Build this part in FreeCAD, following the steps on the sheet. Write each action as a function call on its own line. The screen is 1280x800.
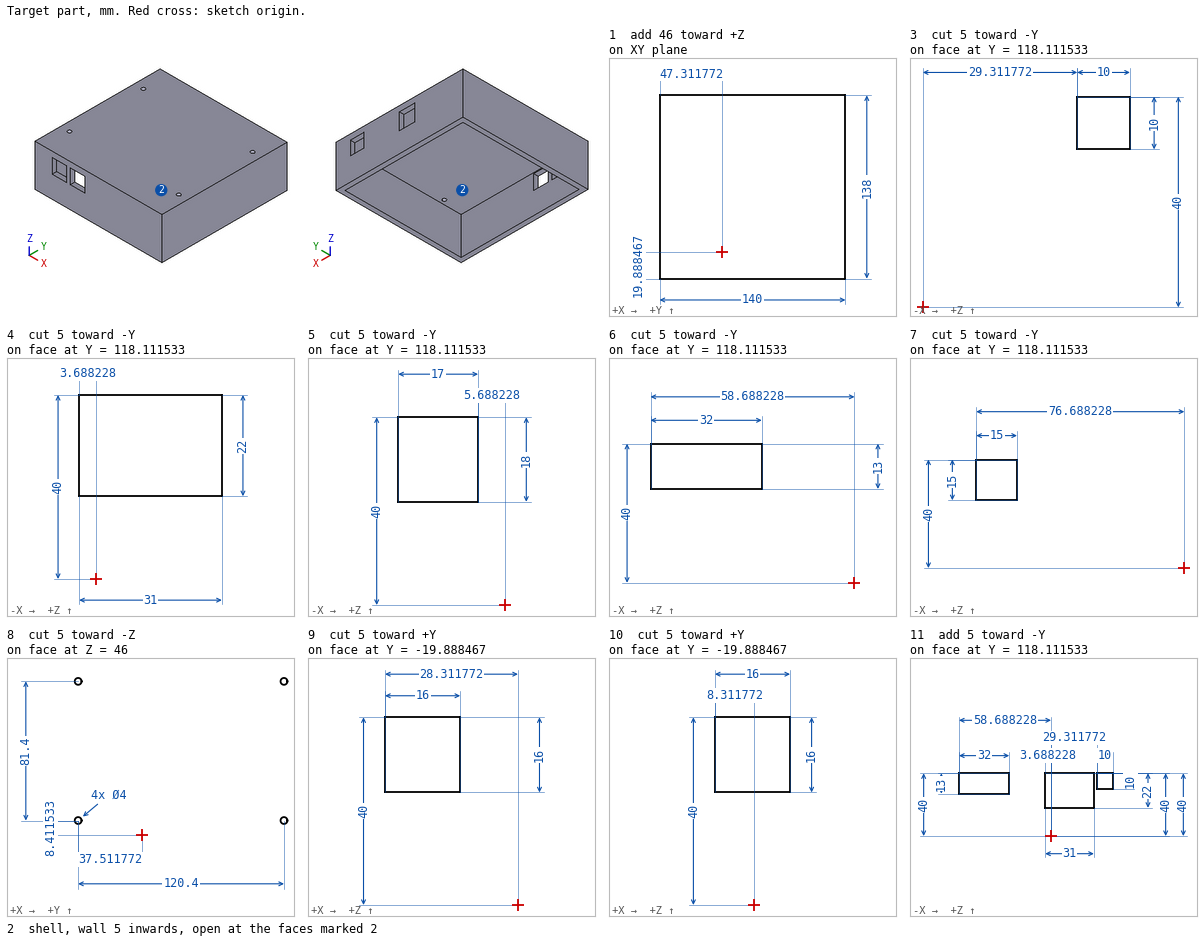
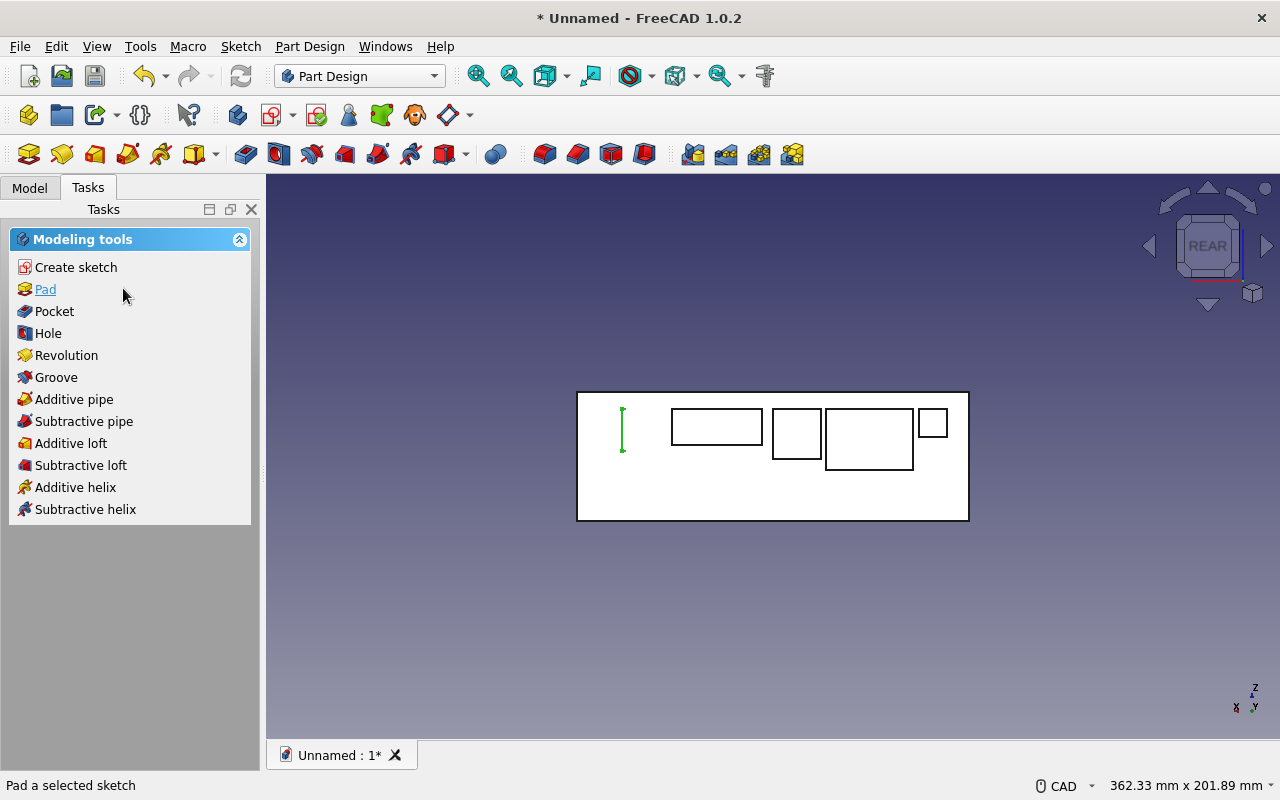
click(246, 154)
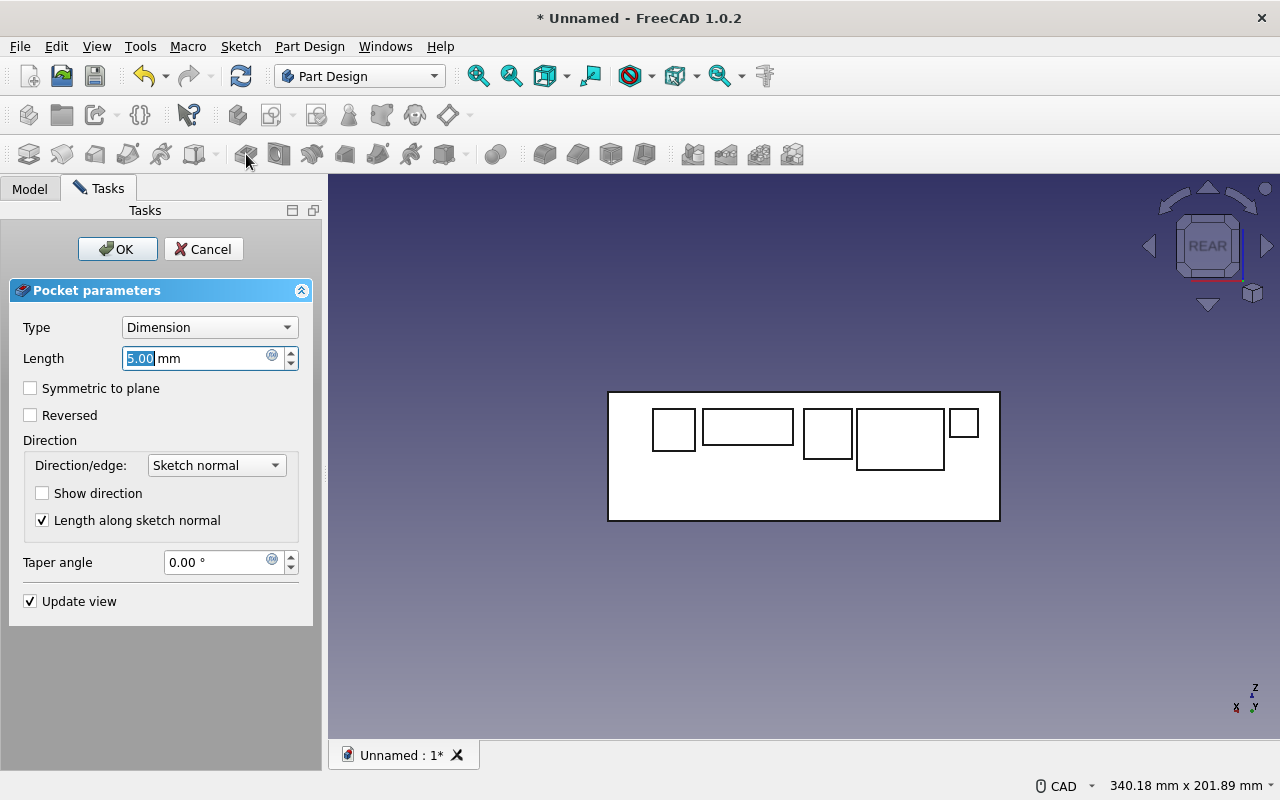
text(5)
key(Tab)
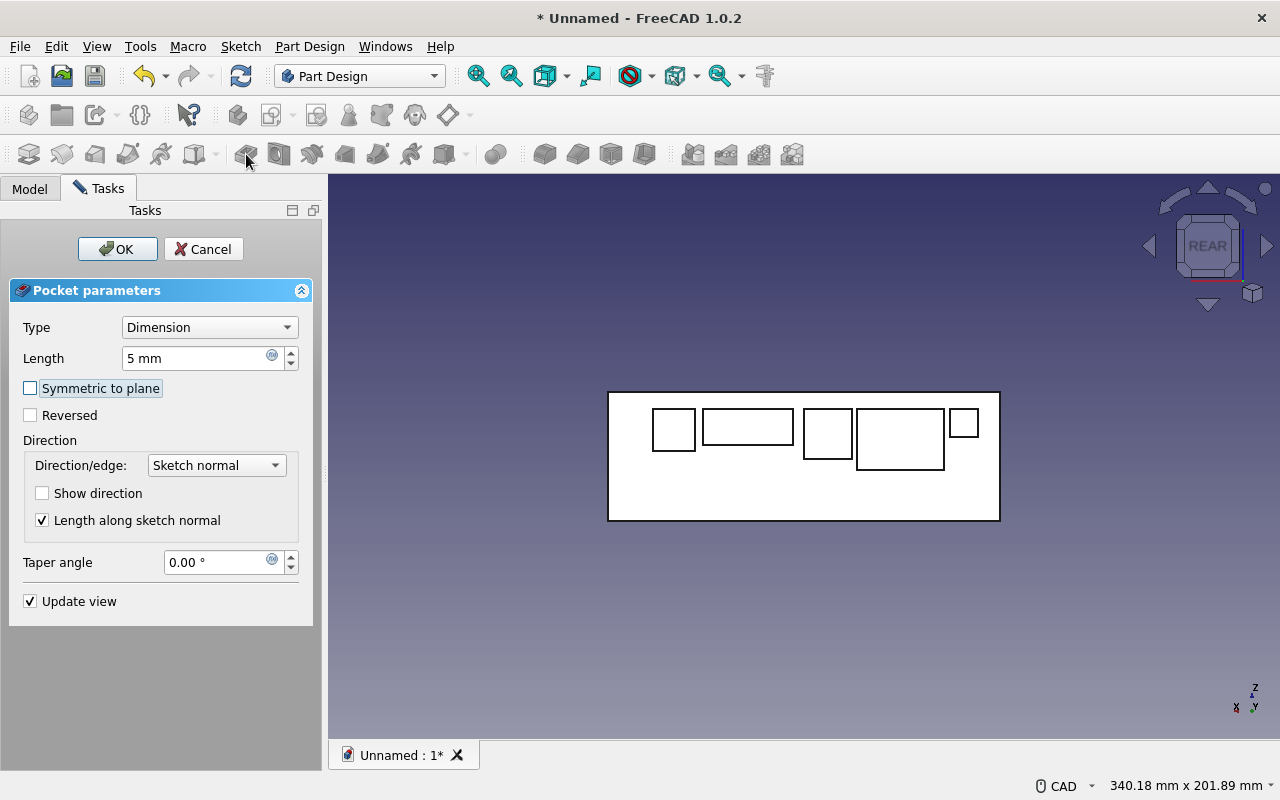
click(118, 249)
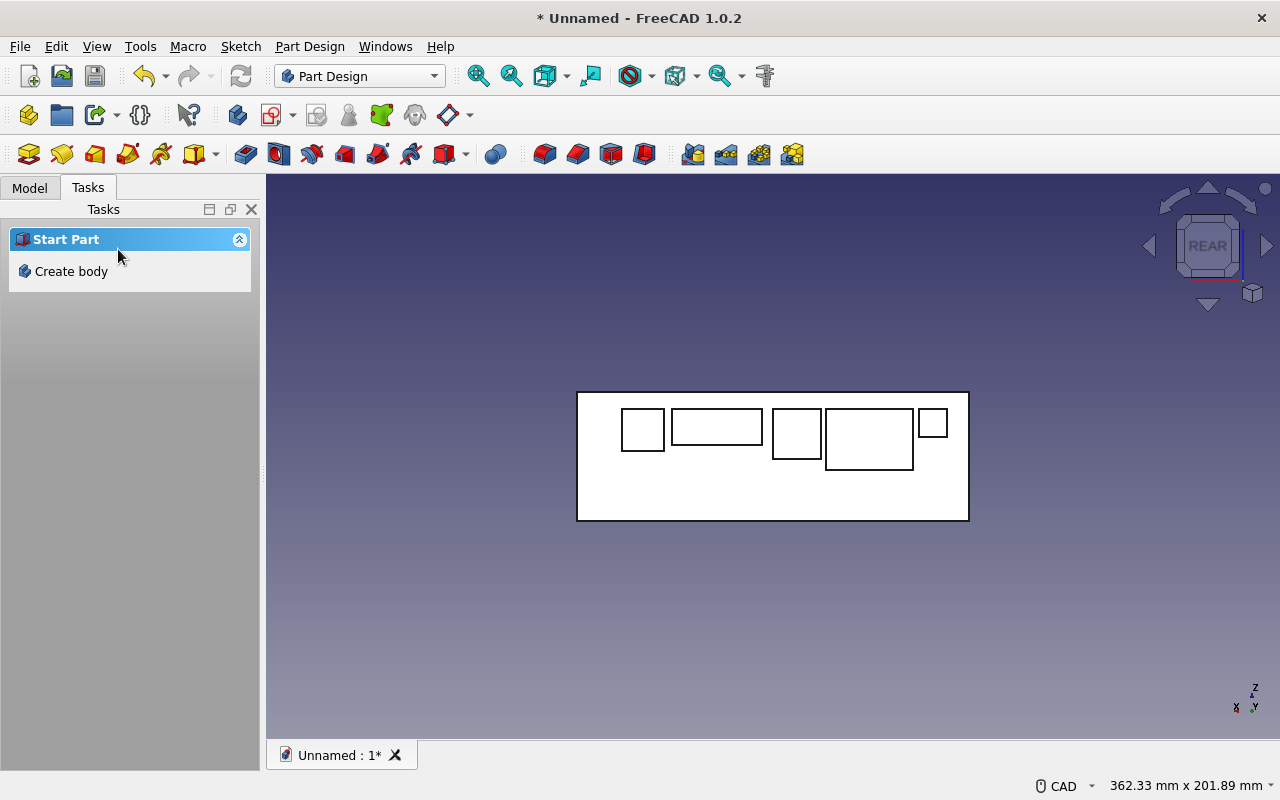
click(479, 76)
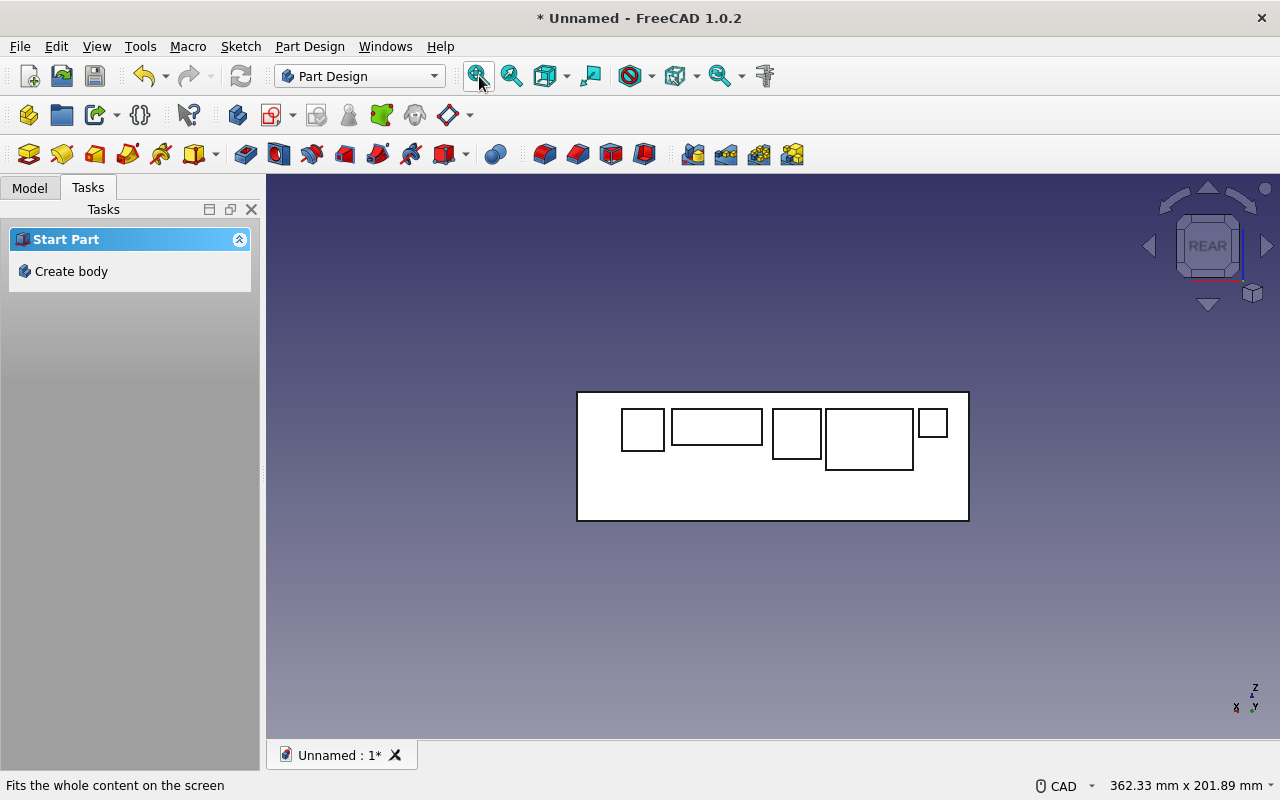
key(0)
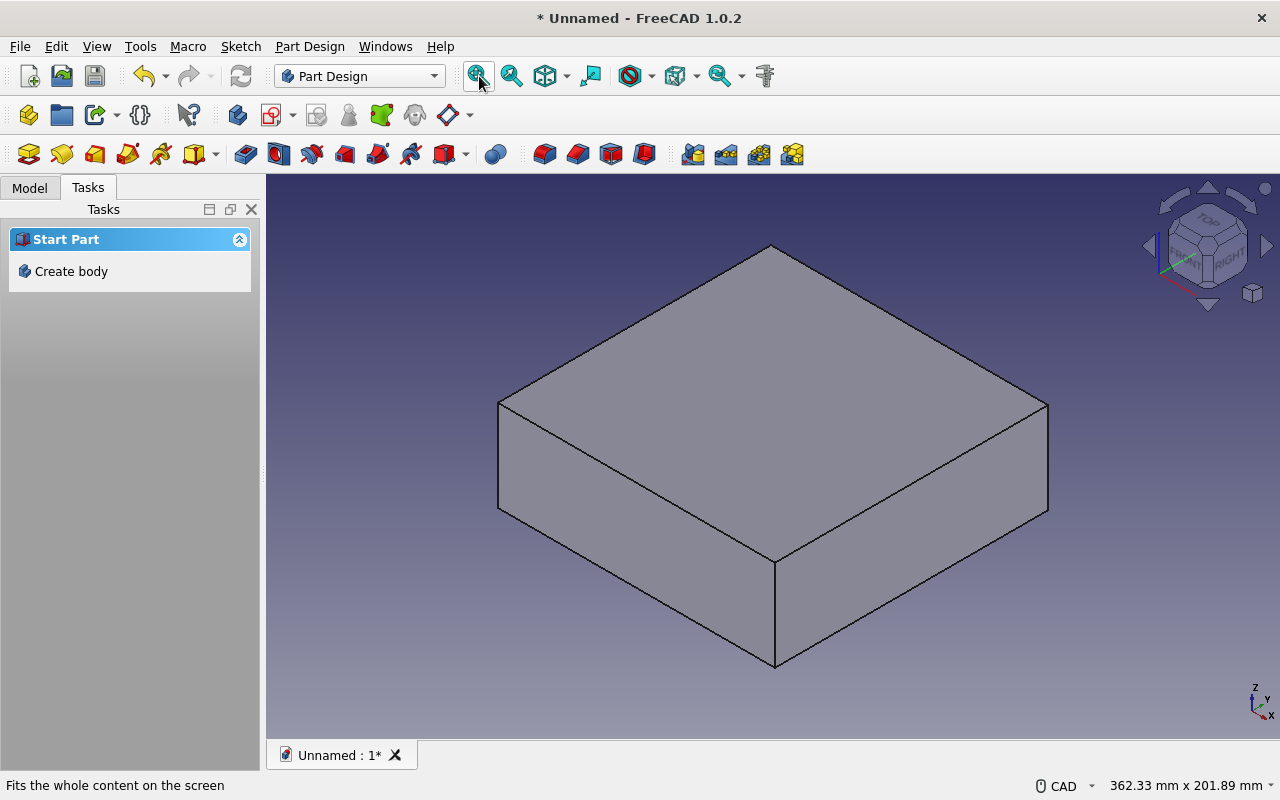
click(773, 403)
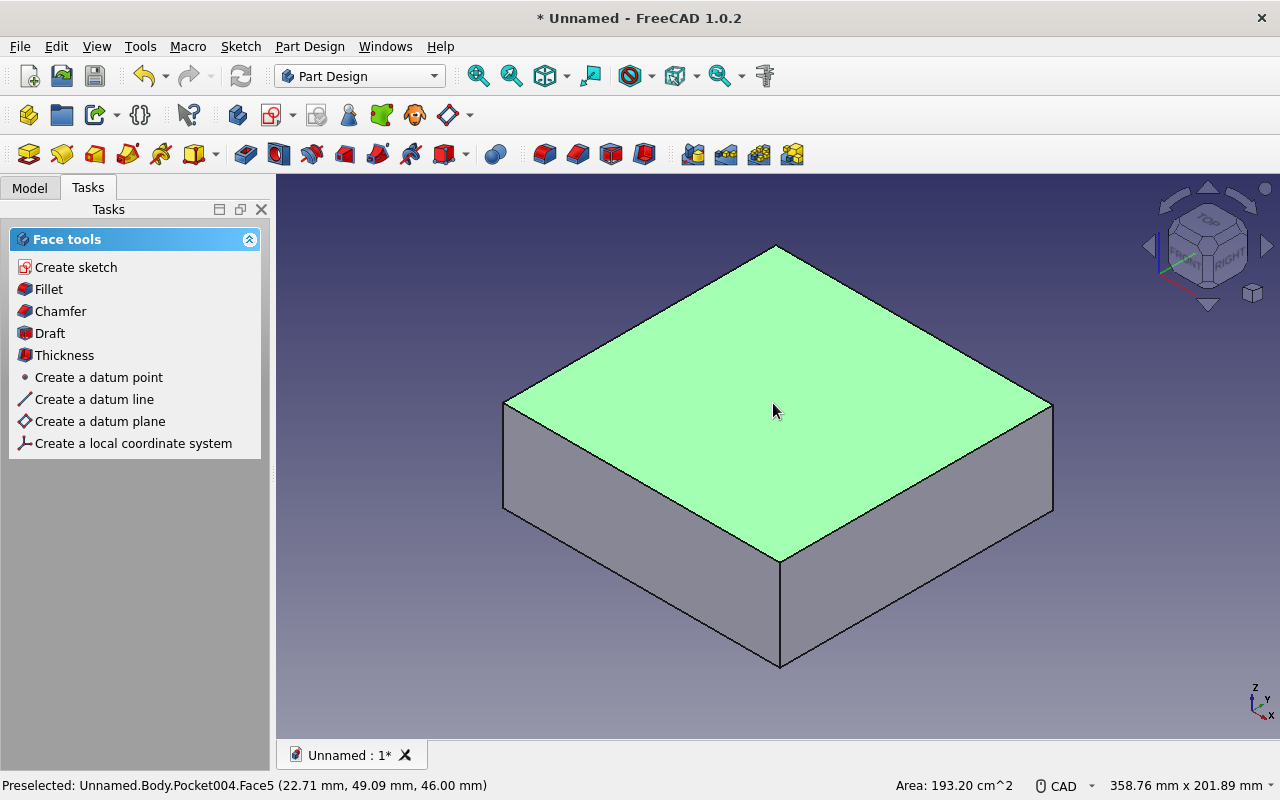
click(270, 116)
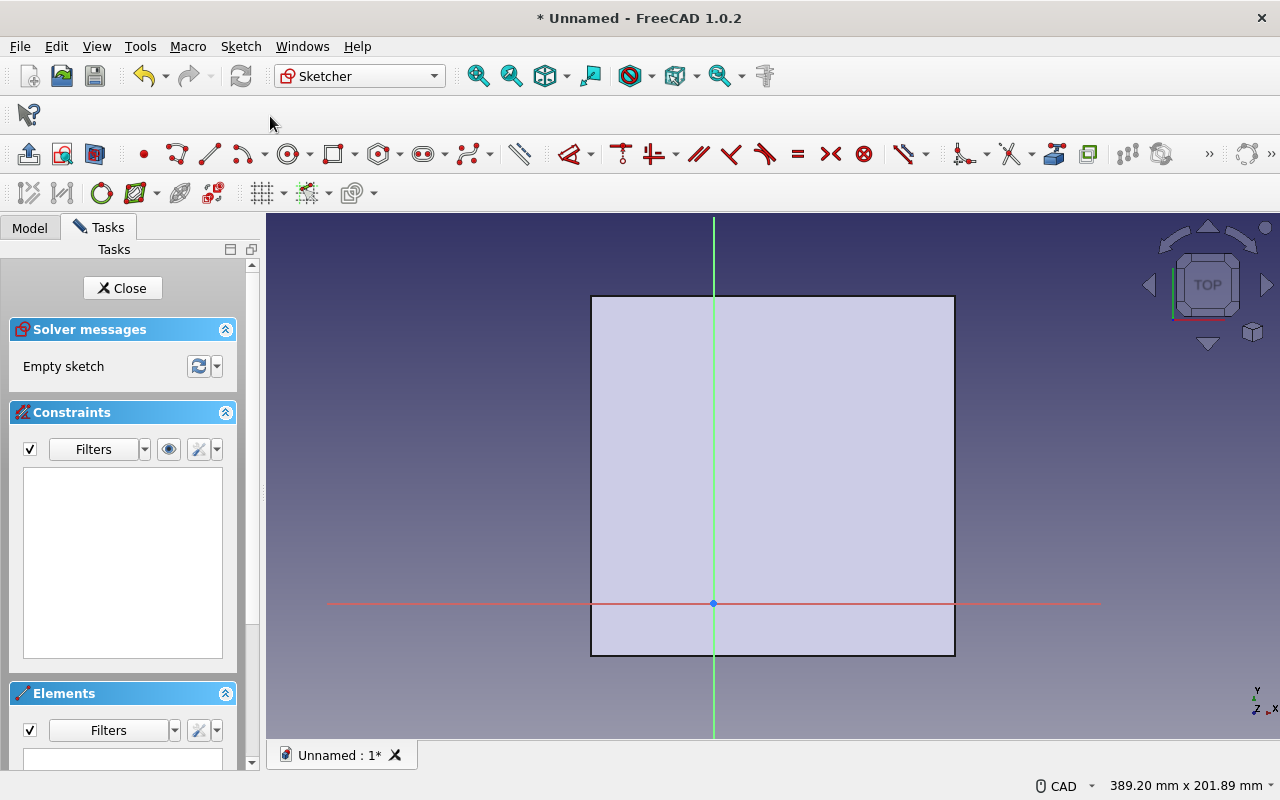
scroll(912, 501, up, 2)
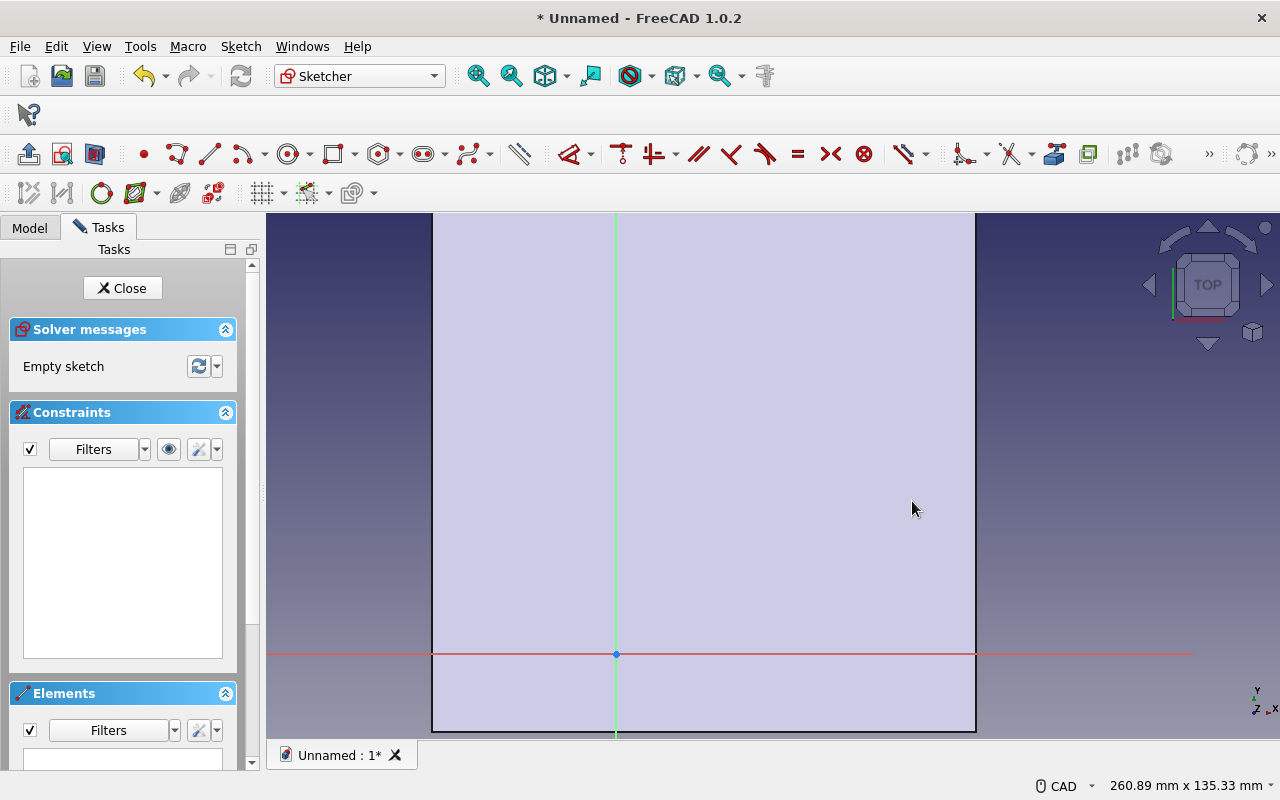
key(g)
key(c)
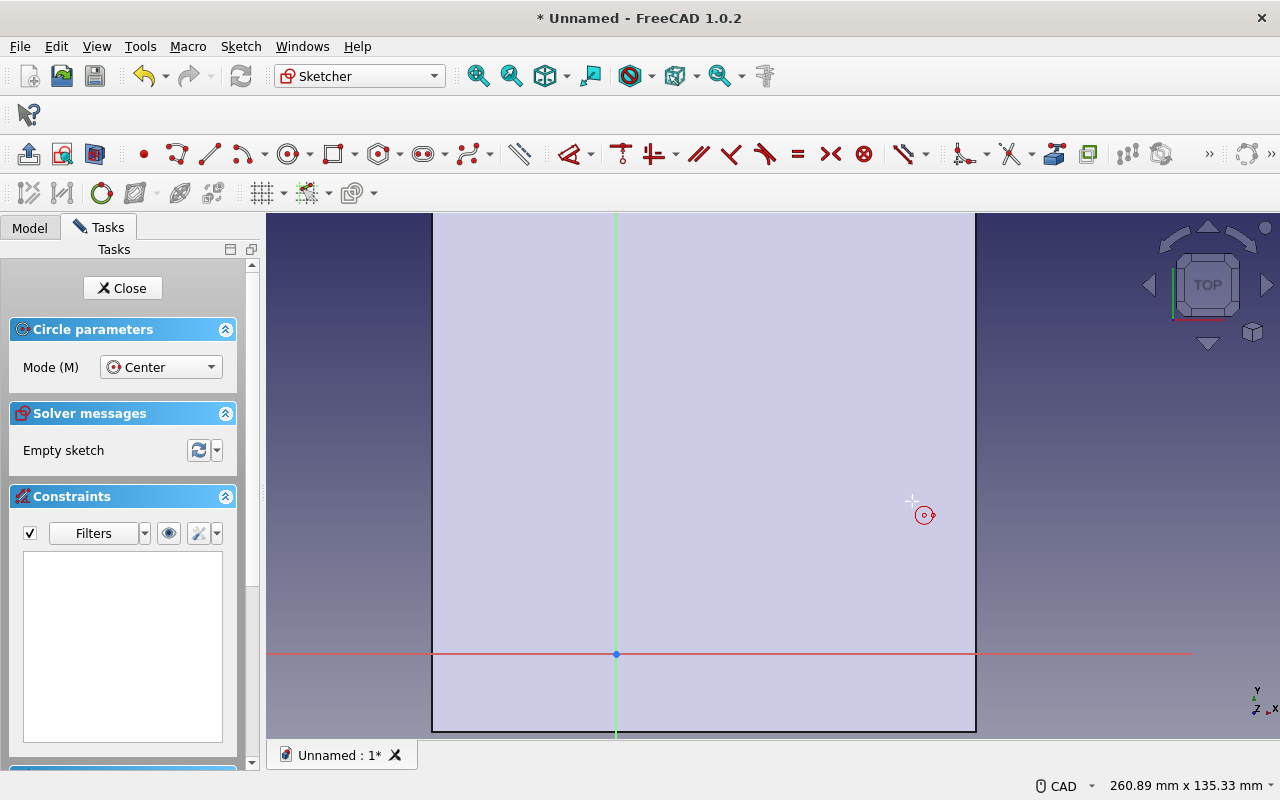
scroll(470, 622, up, 6)